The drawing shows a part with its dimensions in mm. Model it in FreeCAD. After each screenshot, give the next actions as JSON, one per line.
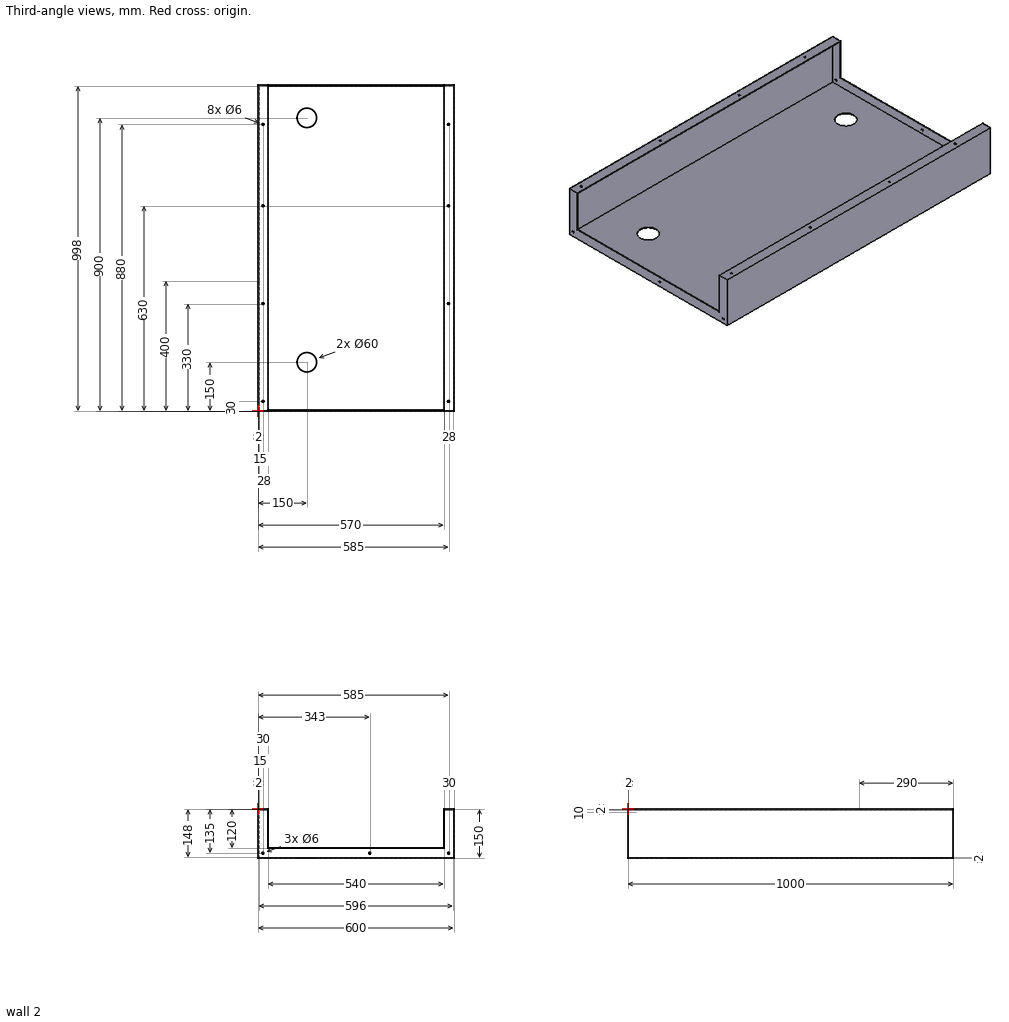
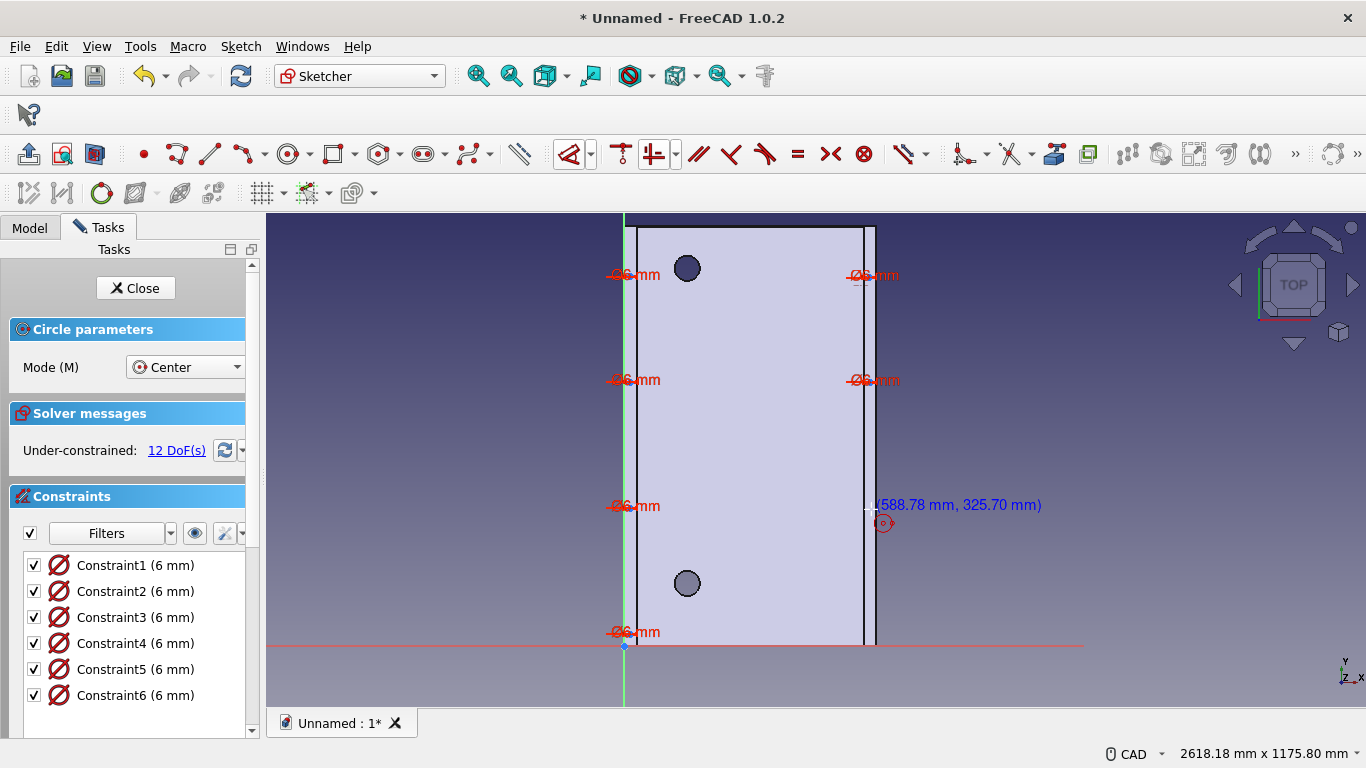
{"action": "left_click", "coordinate": [870, 508]}
{"action": "mouse_move", "coordinate": [871, 507]}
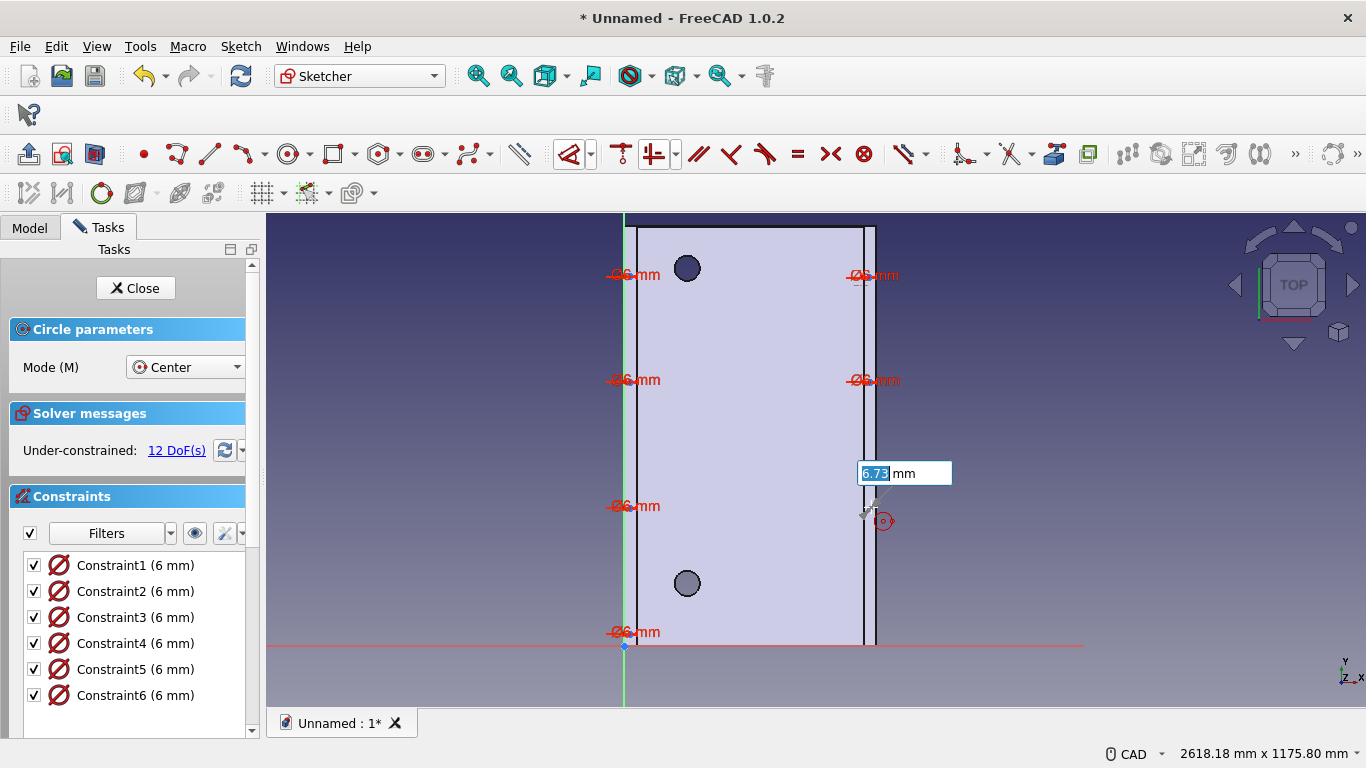
{"action": "type", "text": "6"}
{"action": "key", "text": "Return"}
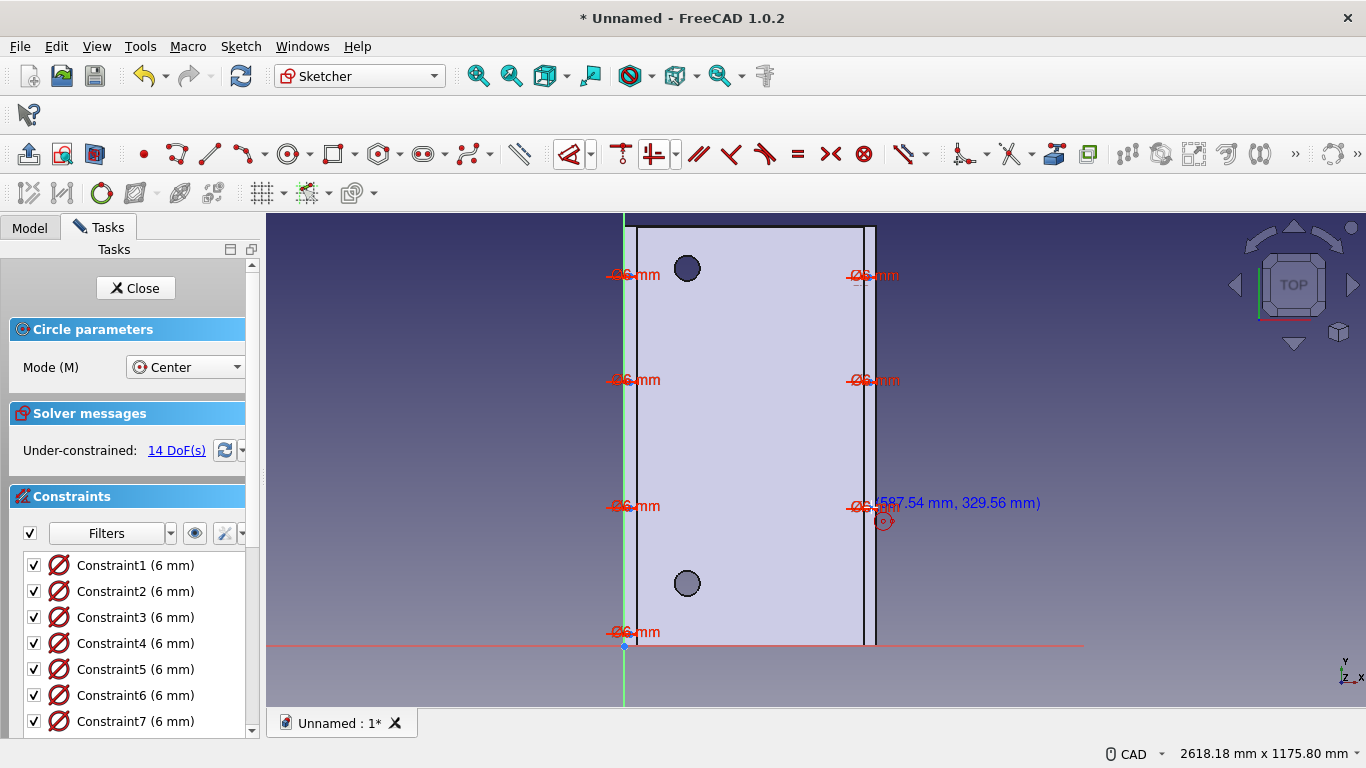
{"action": "scroll", "coordinate": [870, 634], "scroll_direction": "up", "scroll_amount": 15}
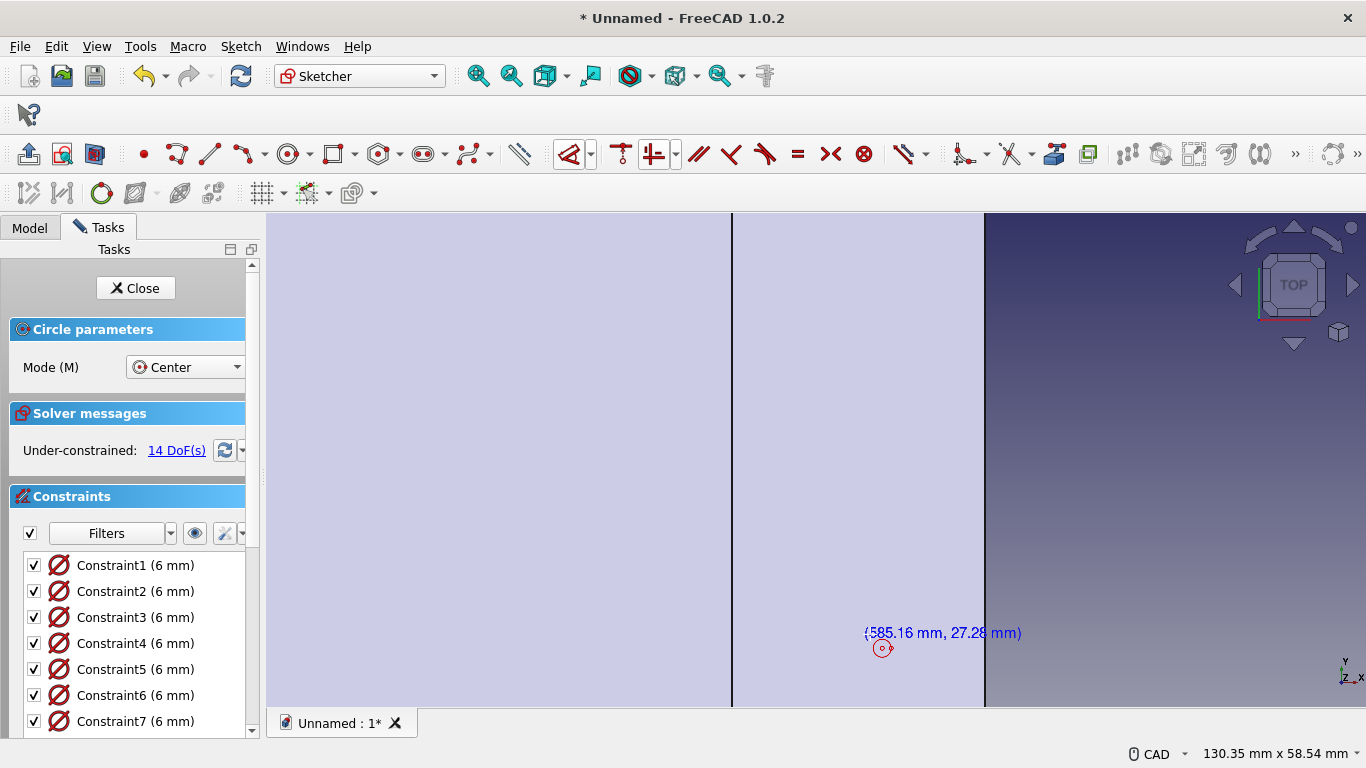
{"action": "scroll", "coordinate": [870, 634], "scroll_direction": "down", "scroll_amount": 15}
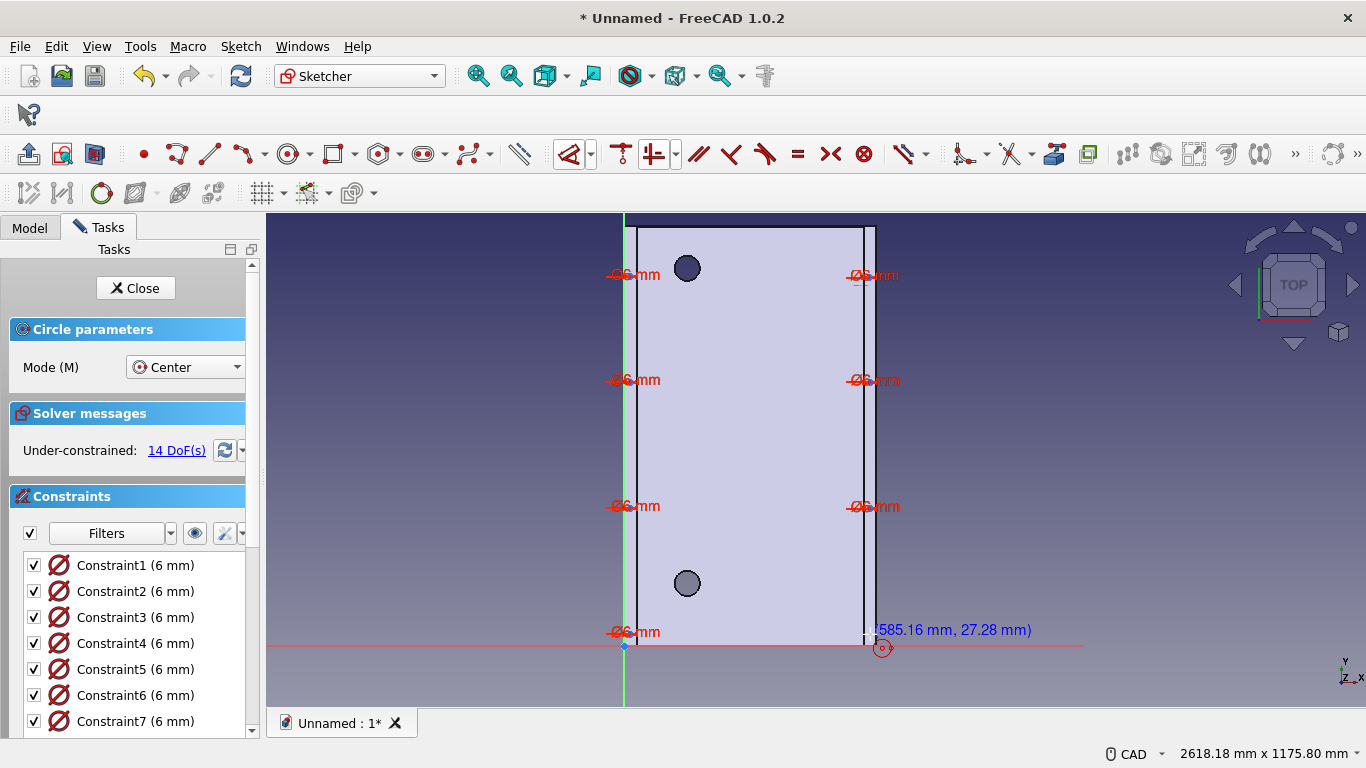
{"action": "scroll", "coordinate": [870, 634], "scroll_direction": "up", "scroll_amount": 2}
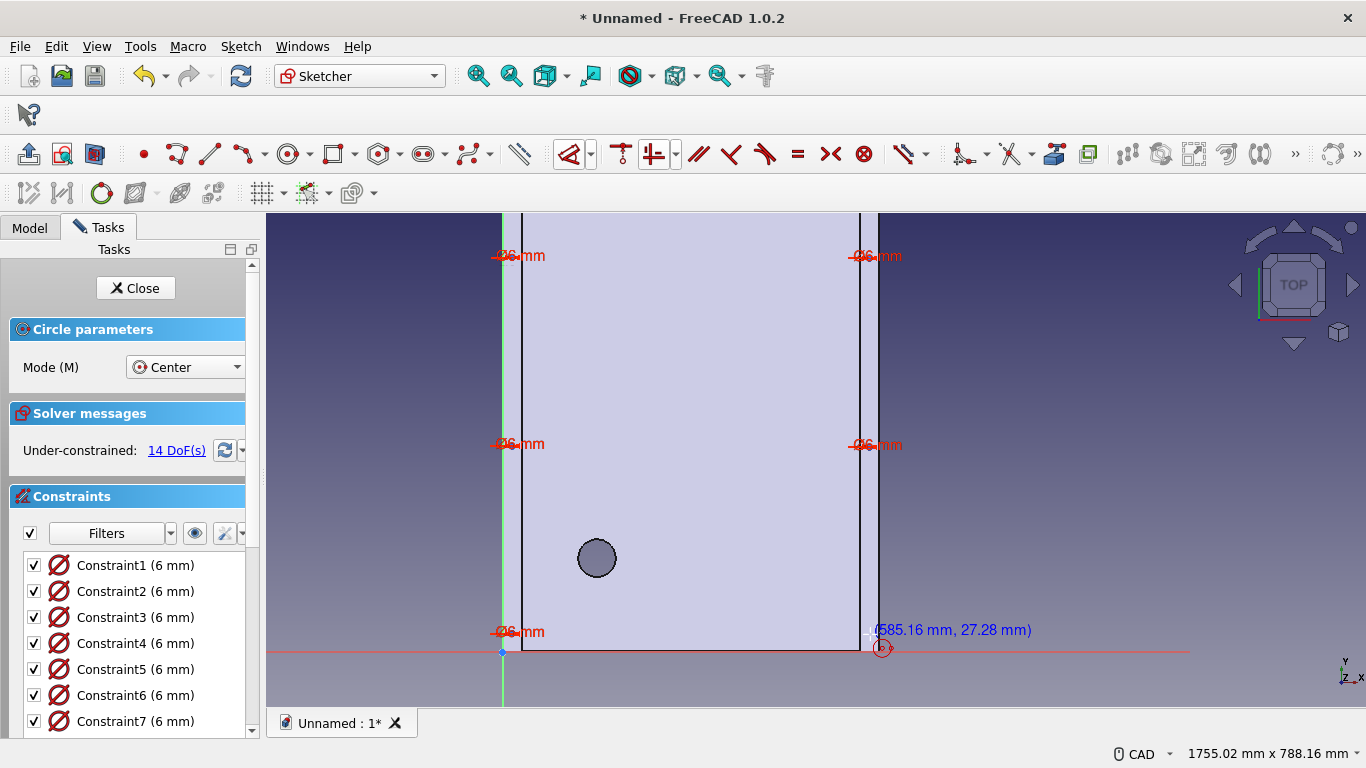
{"action": "left_click", "coordinate": [870, 633]}
{"action": "mouse_move", "coordinate": [871, 632]}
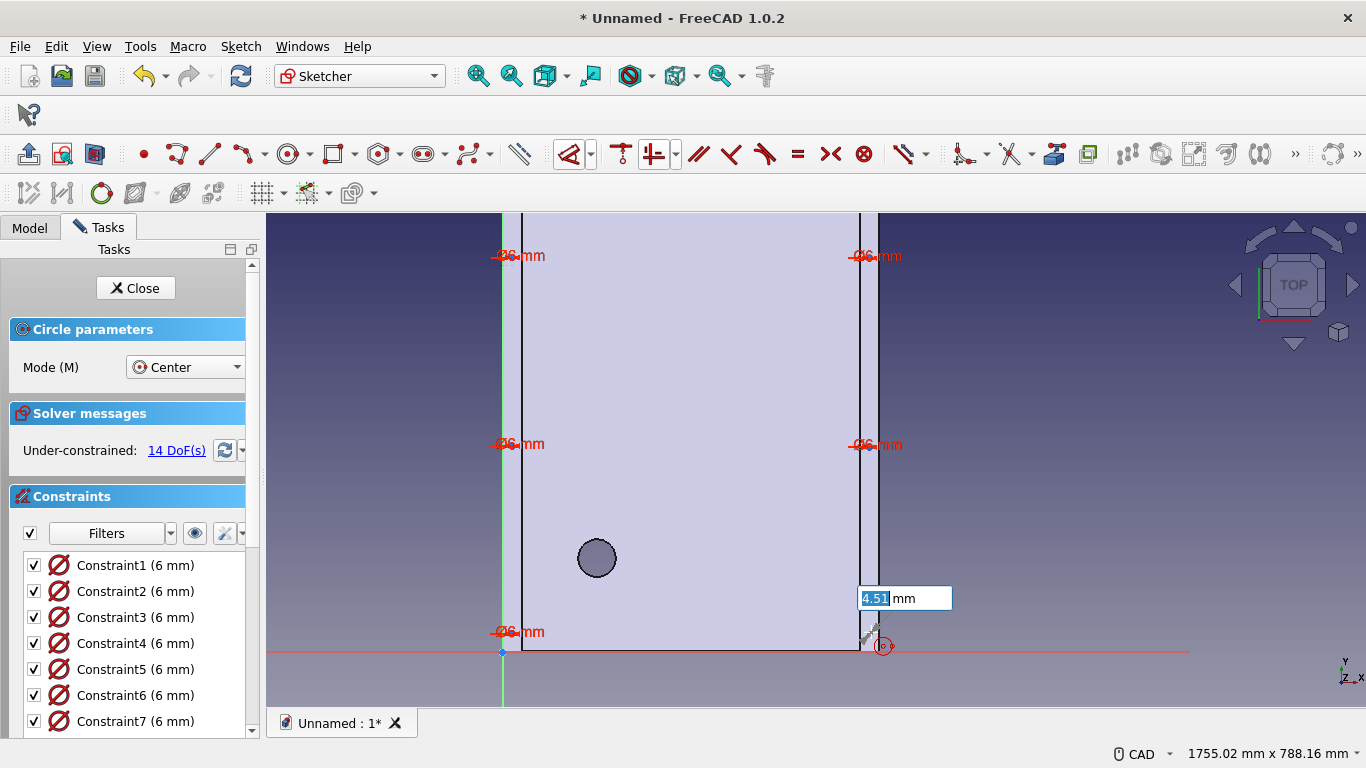
{"action": "type", "text": "6"}
{"action": "key", "text": "Return"}
{"action": "key", "text": "Escape"}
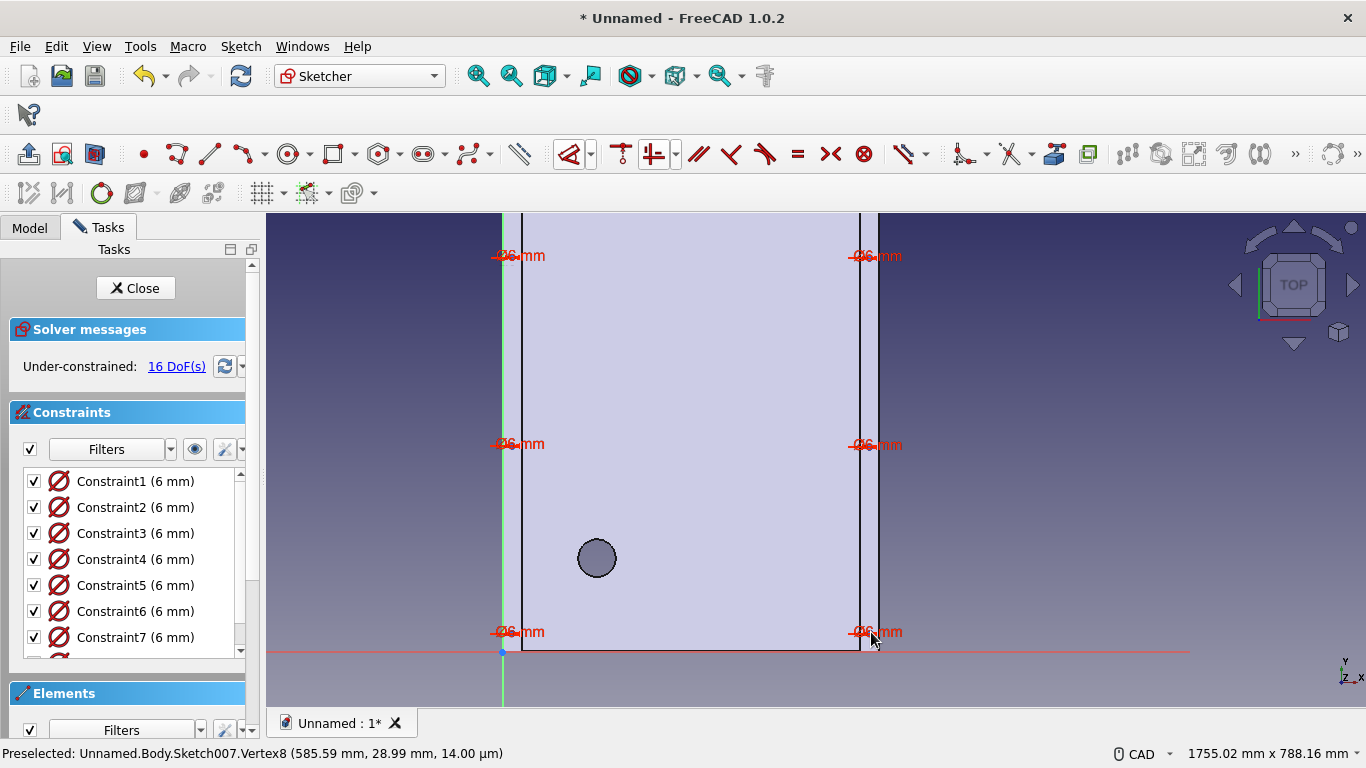
{"action": "scroll", "coordinate": [821, 563], "scroll_direction": "down", "scroll_amount": 3}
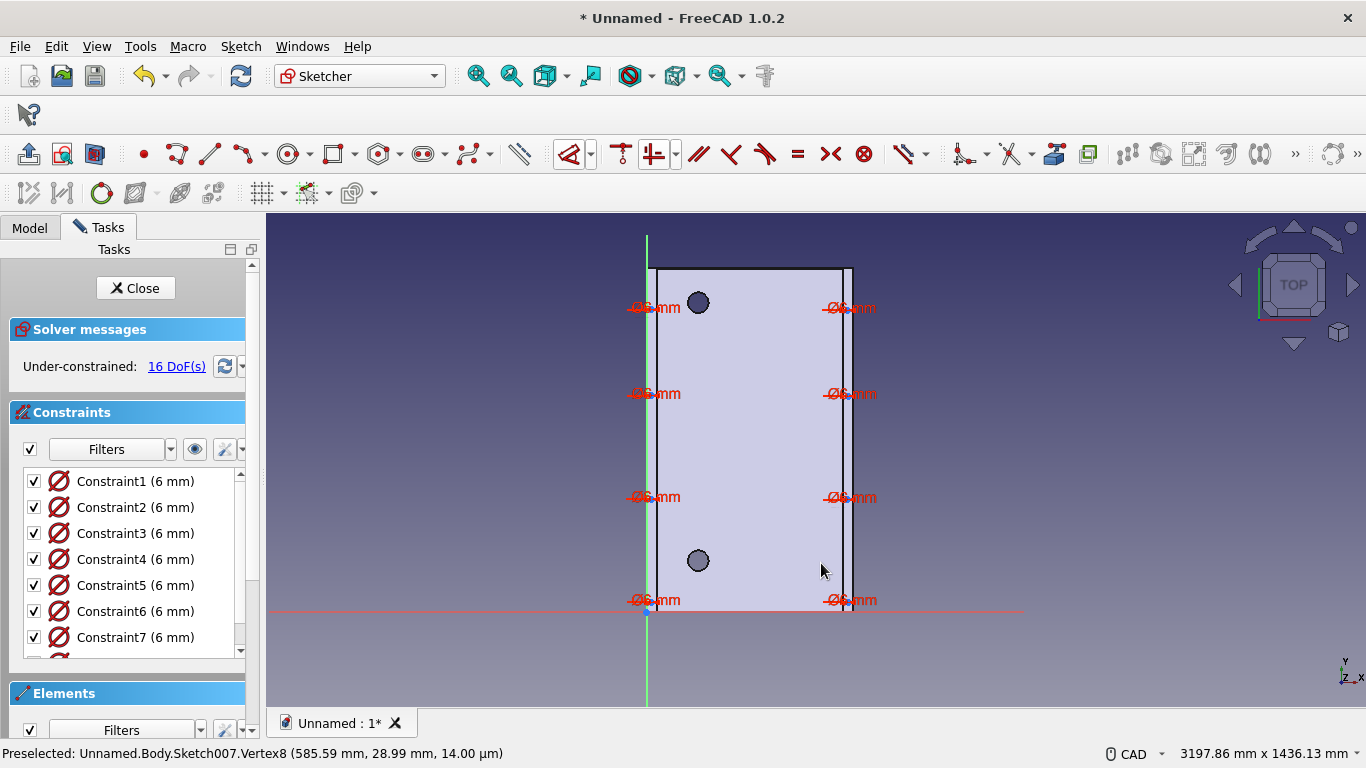
{"action": "scroll", "coordinate": [652, 310], "scroll_direction": "up", "scroll_amount": 11}